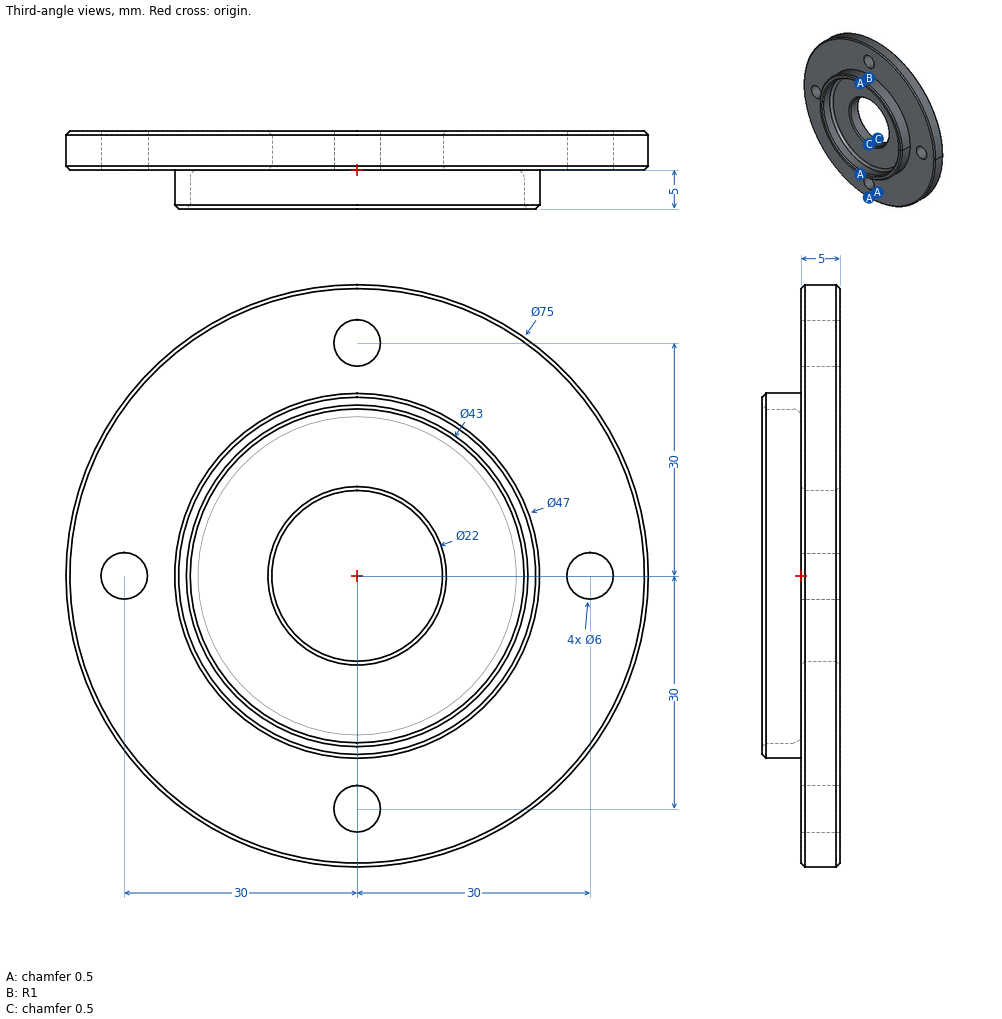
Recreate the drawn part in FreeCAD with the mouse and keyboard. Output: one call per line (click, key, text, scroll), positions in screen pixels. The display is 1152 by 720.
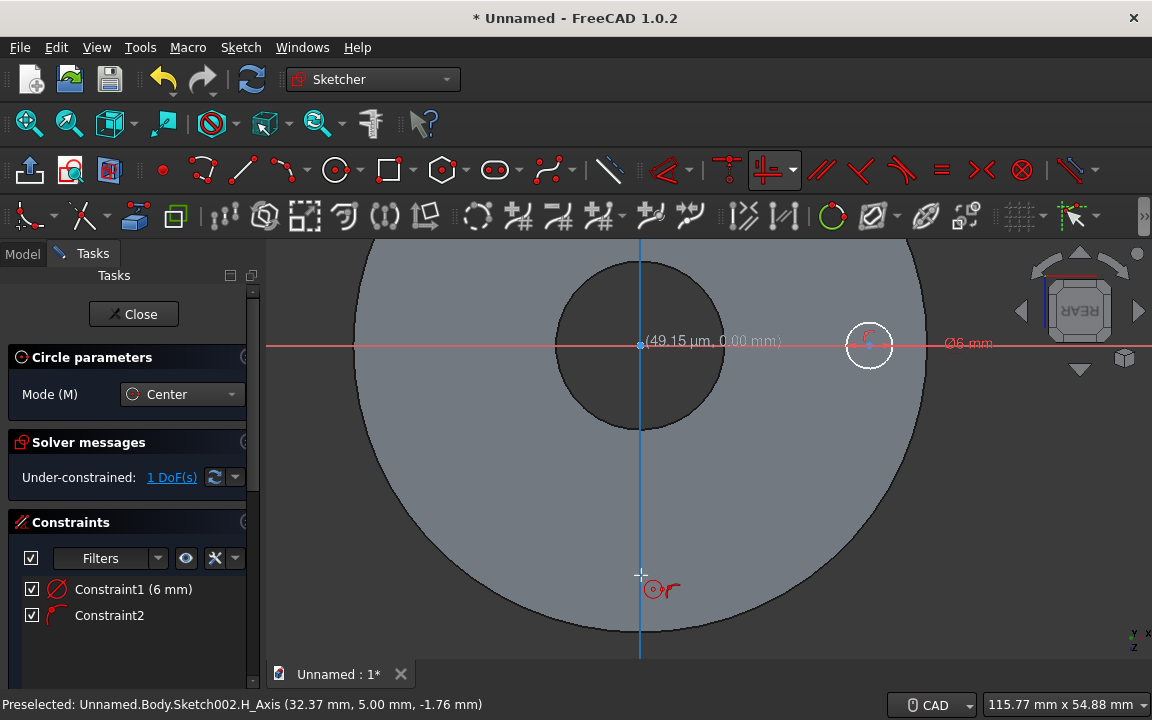
click(640, 575)
move(657, 559)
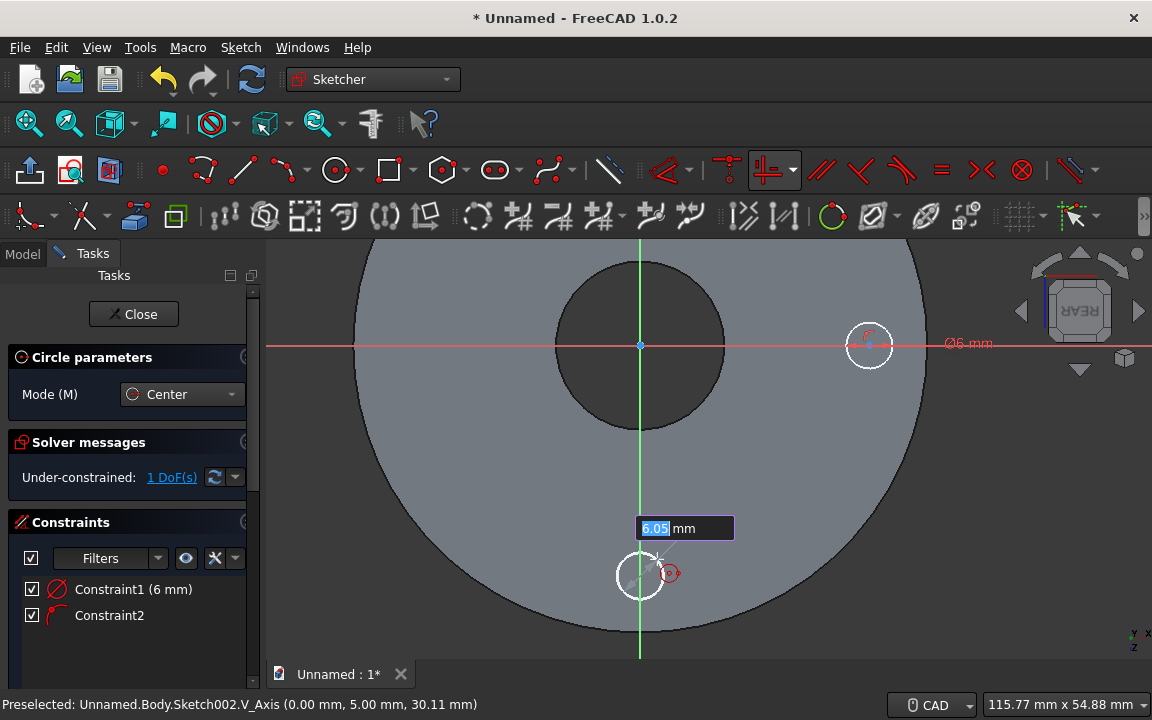
text(6)
key(Return)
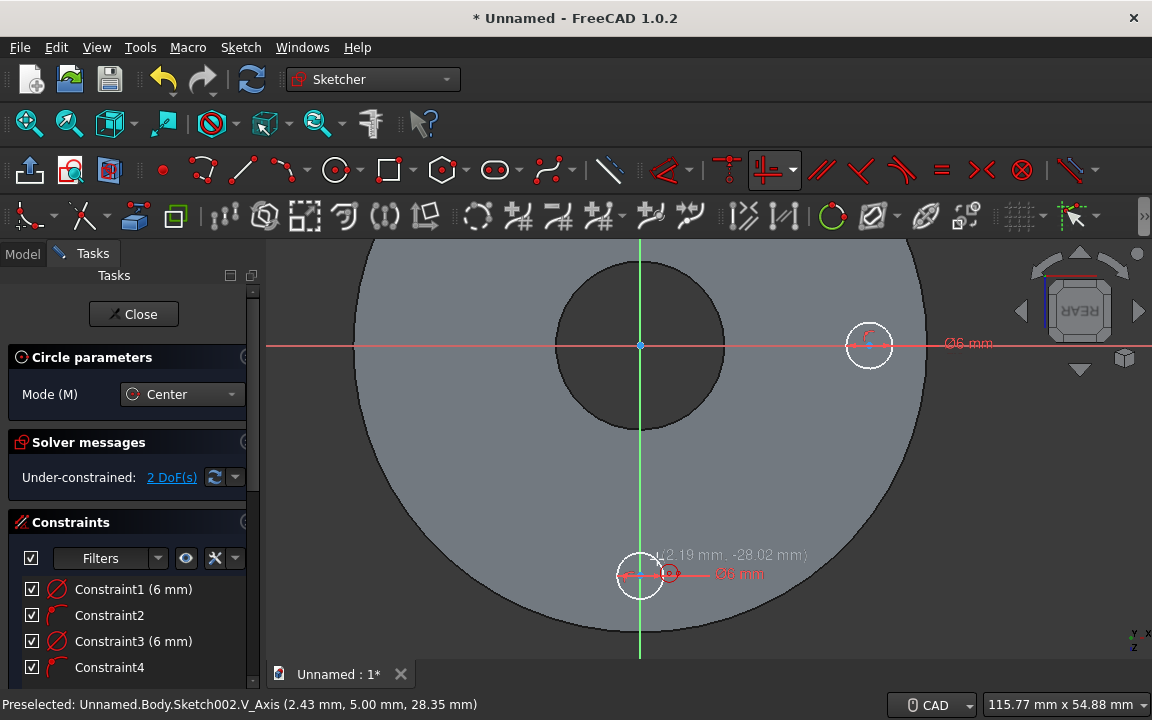
click(411, 346)
move(427, 329)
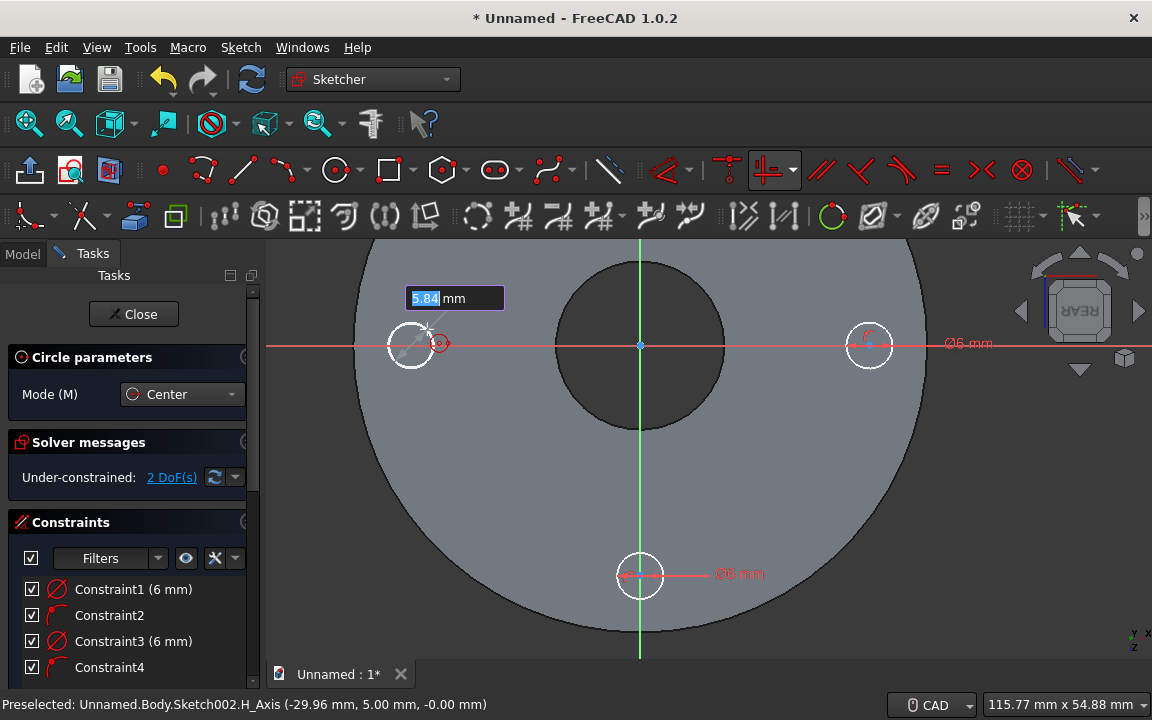
text(6)
key(Return)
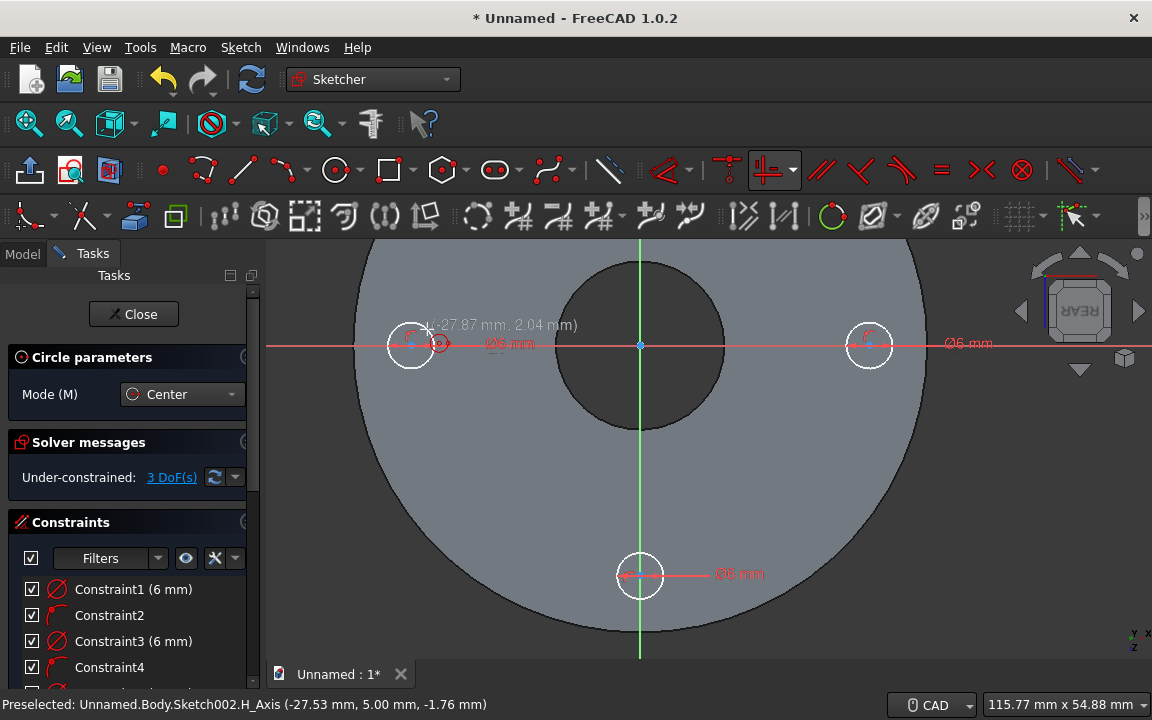
scroll(641, 575, down, 3)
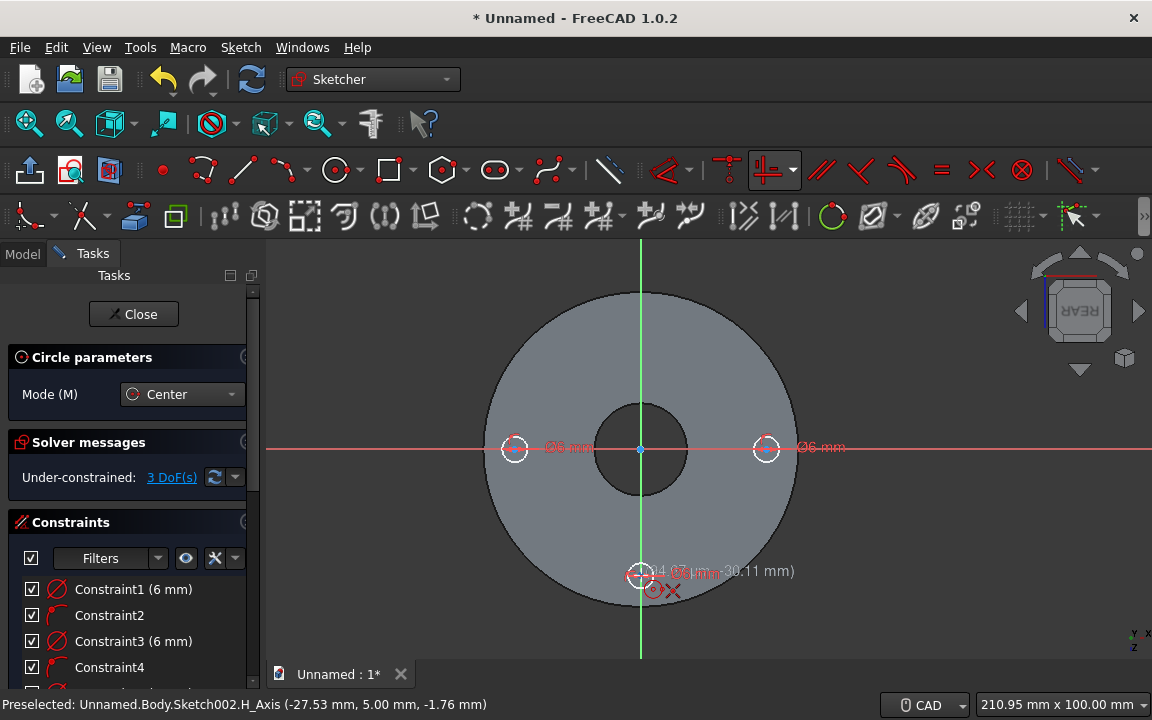
scroll(641, 323, up, 3)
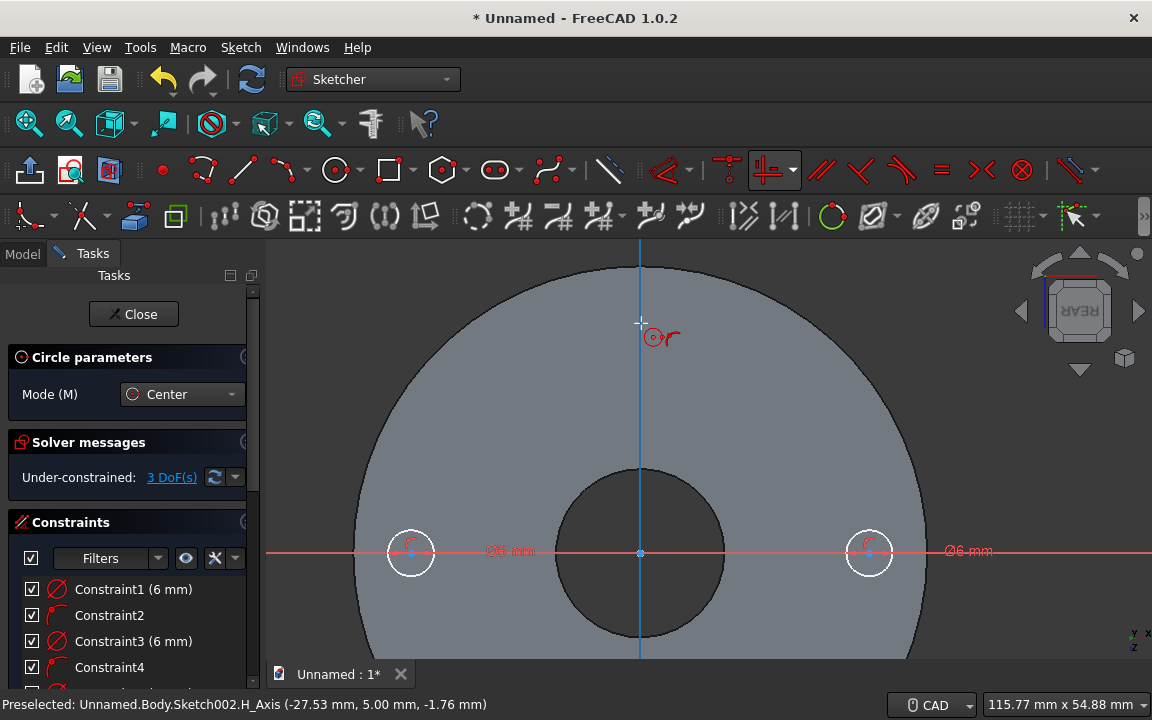
click(640, 324)
move(657, 307)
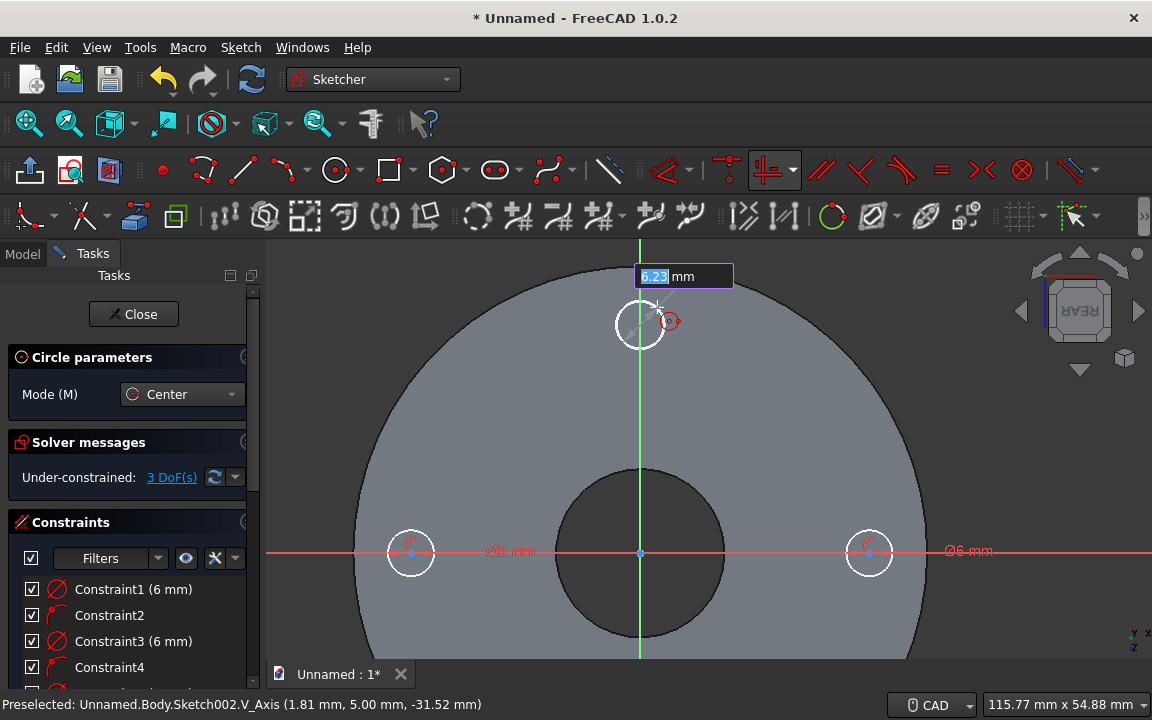
text(6)
key(Return)
key(Escape)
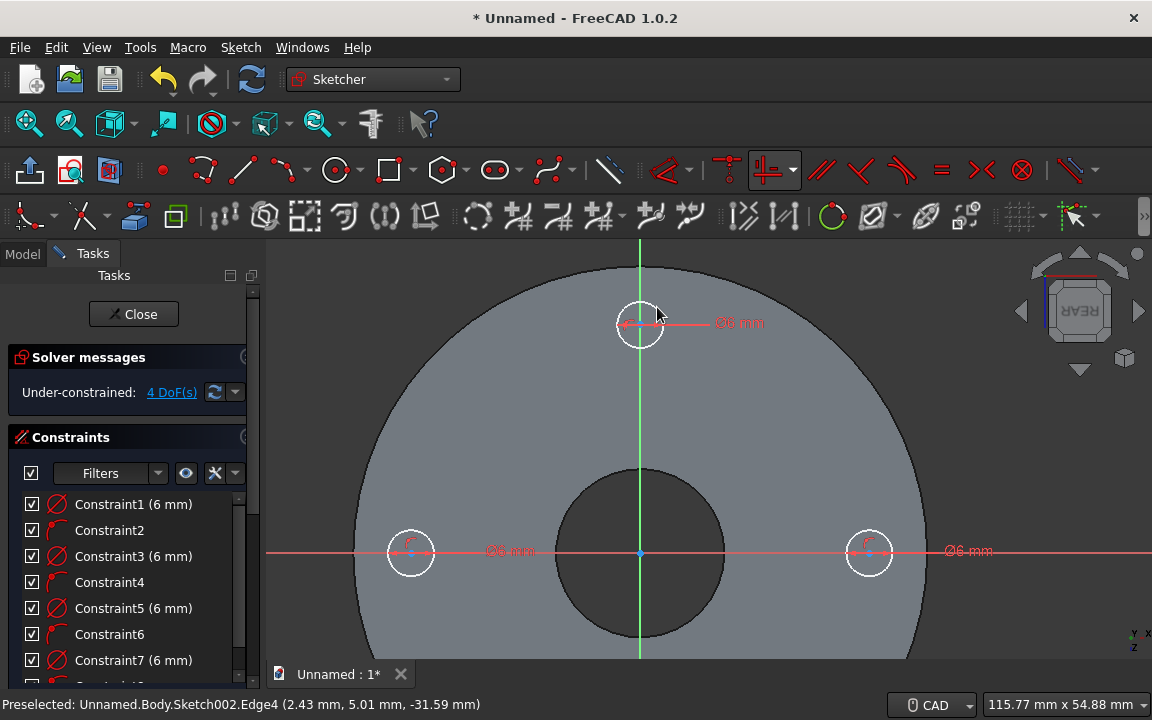
key(d)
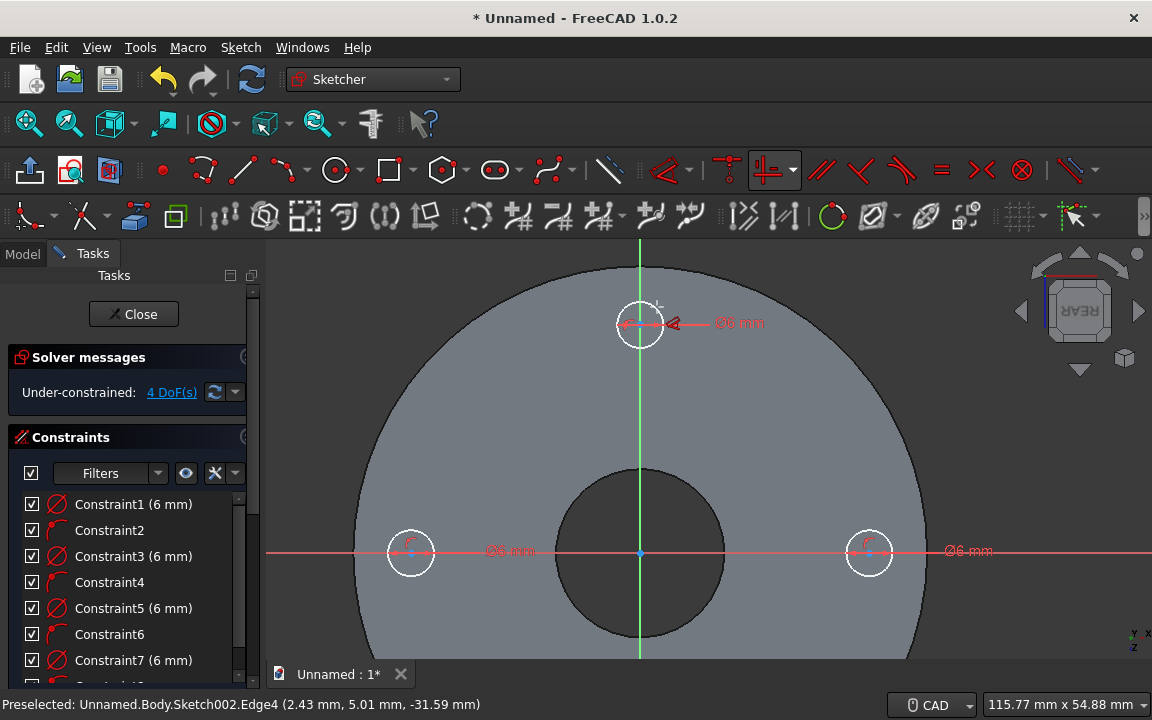
click(869, 553)
click(755, 587)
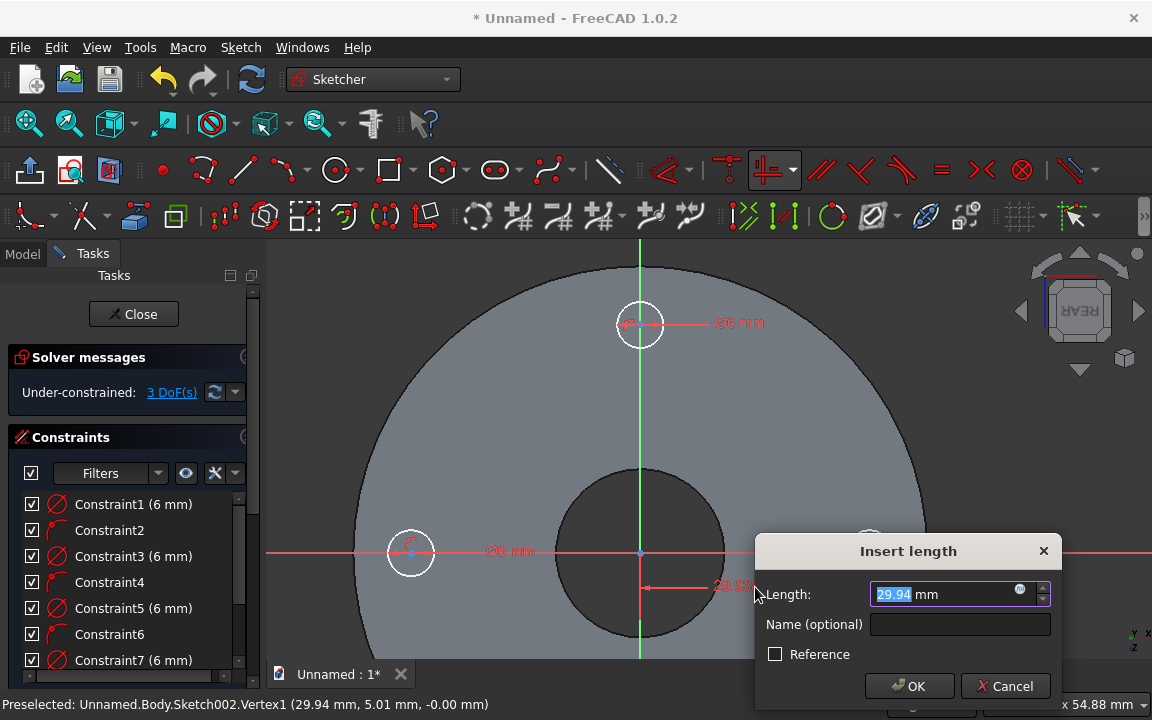
text(30)
key(Return)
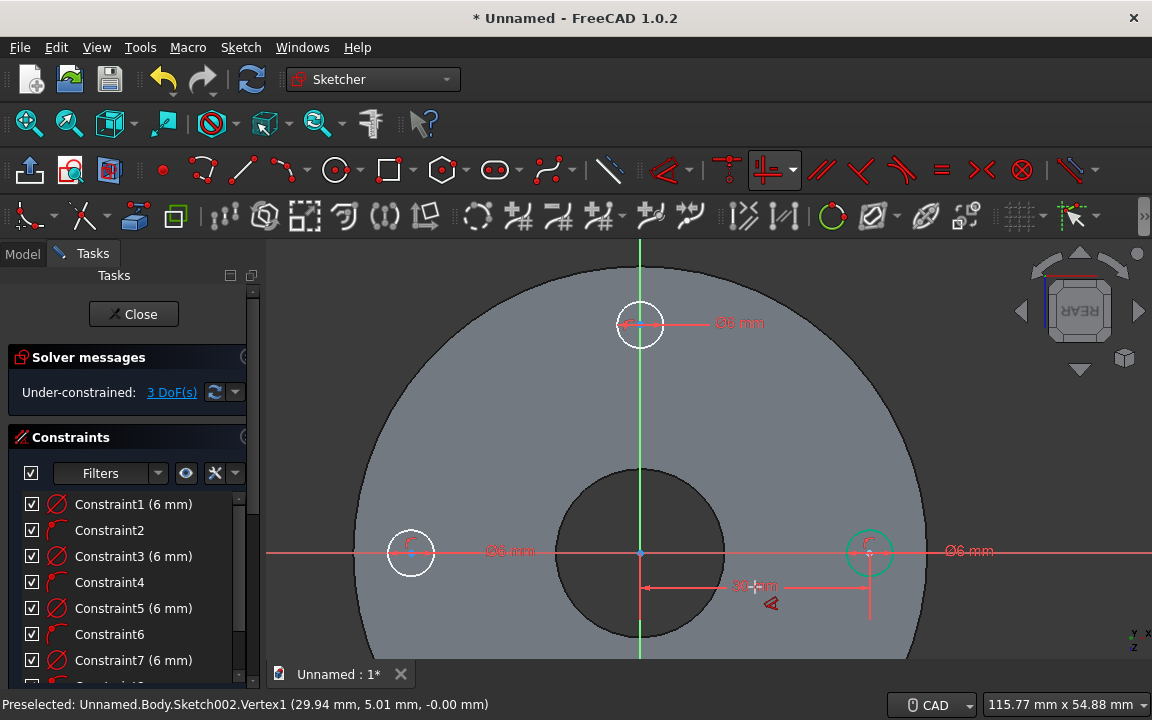
scroll(641, 322, down, 3)